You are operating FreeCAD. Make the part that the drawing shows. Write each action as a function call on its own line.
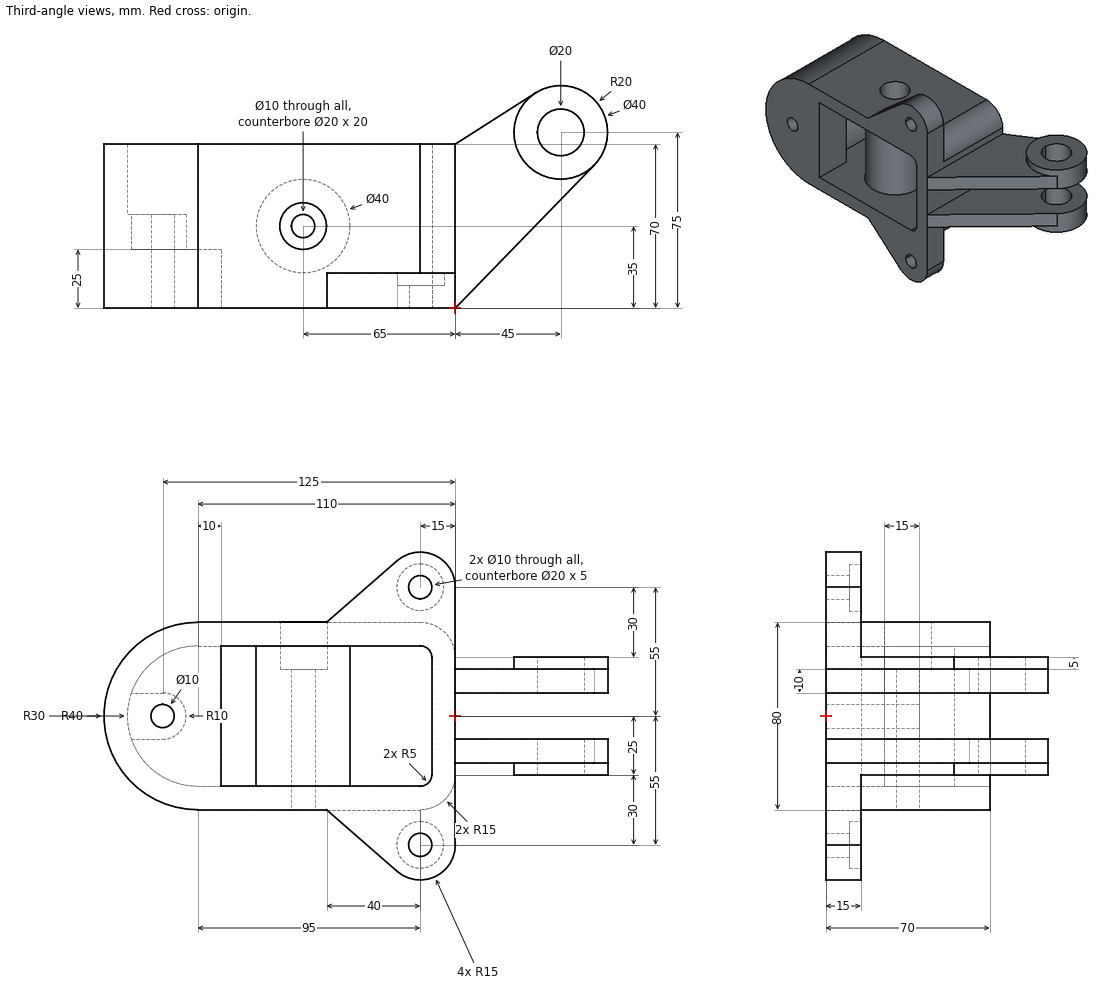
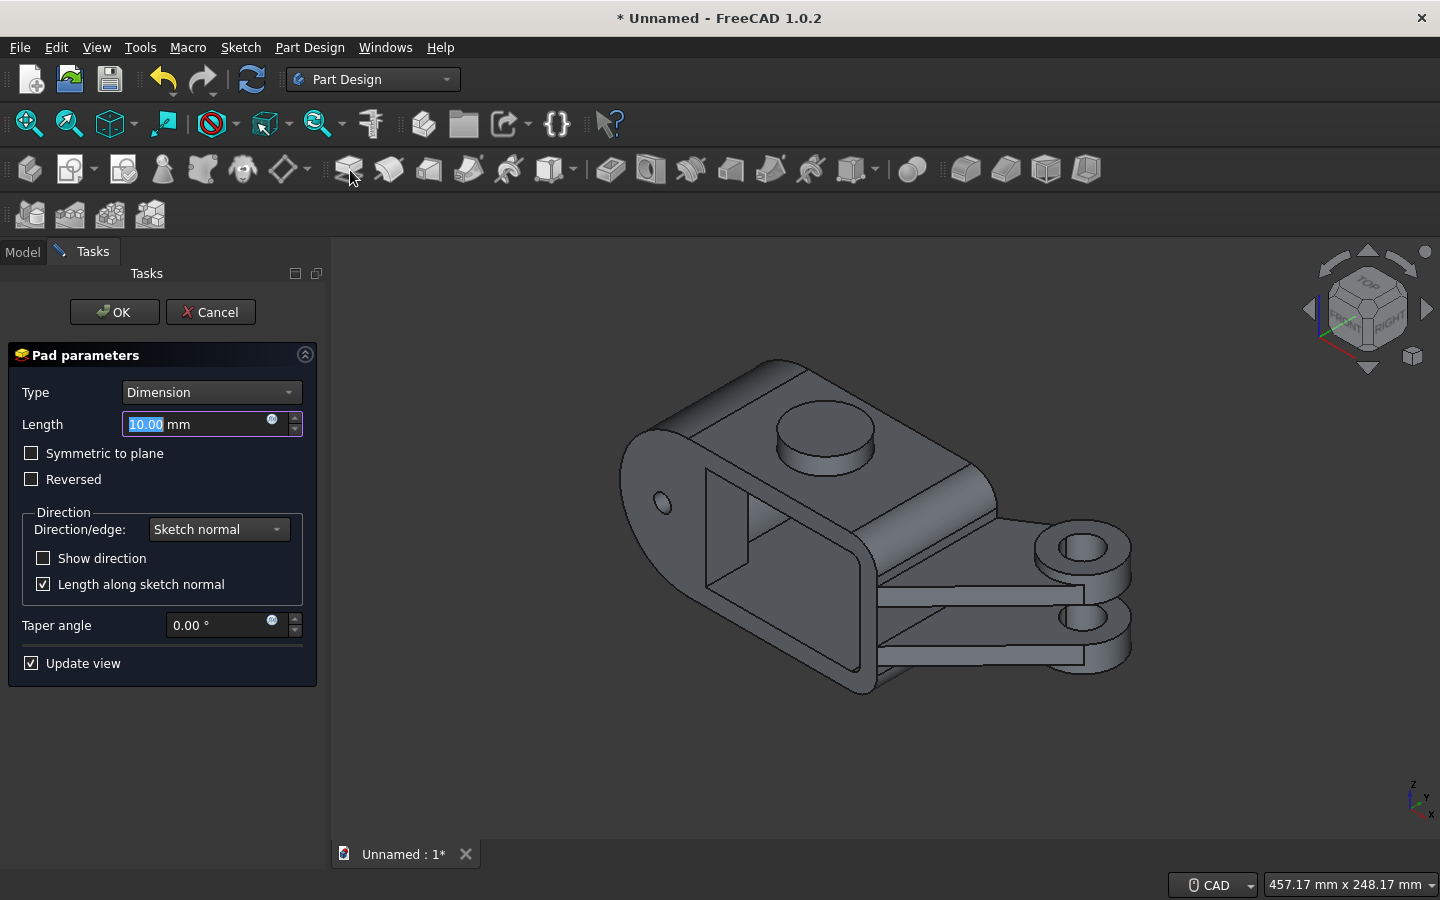
text(80)
key(Tab)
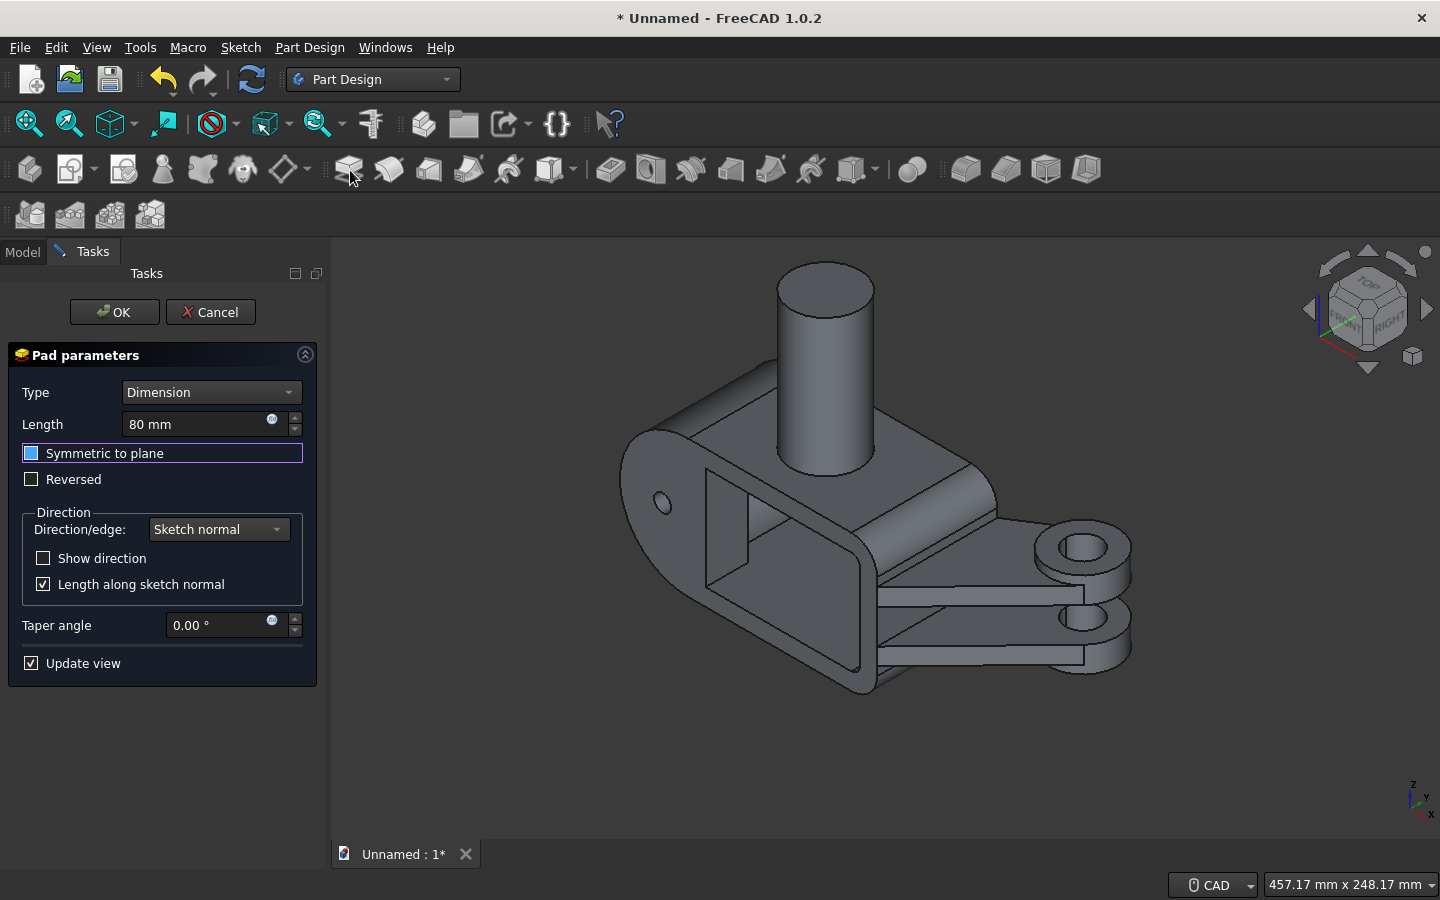
click(30, 479)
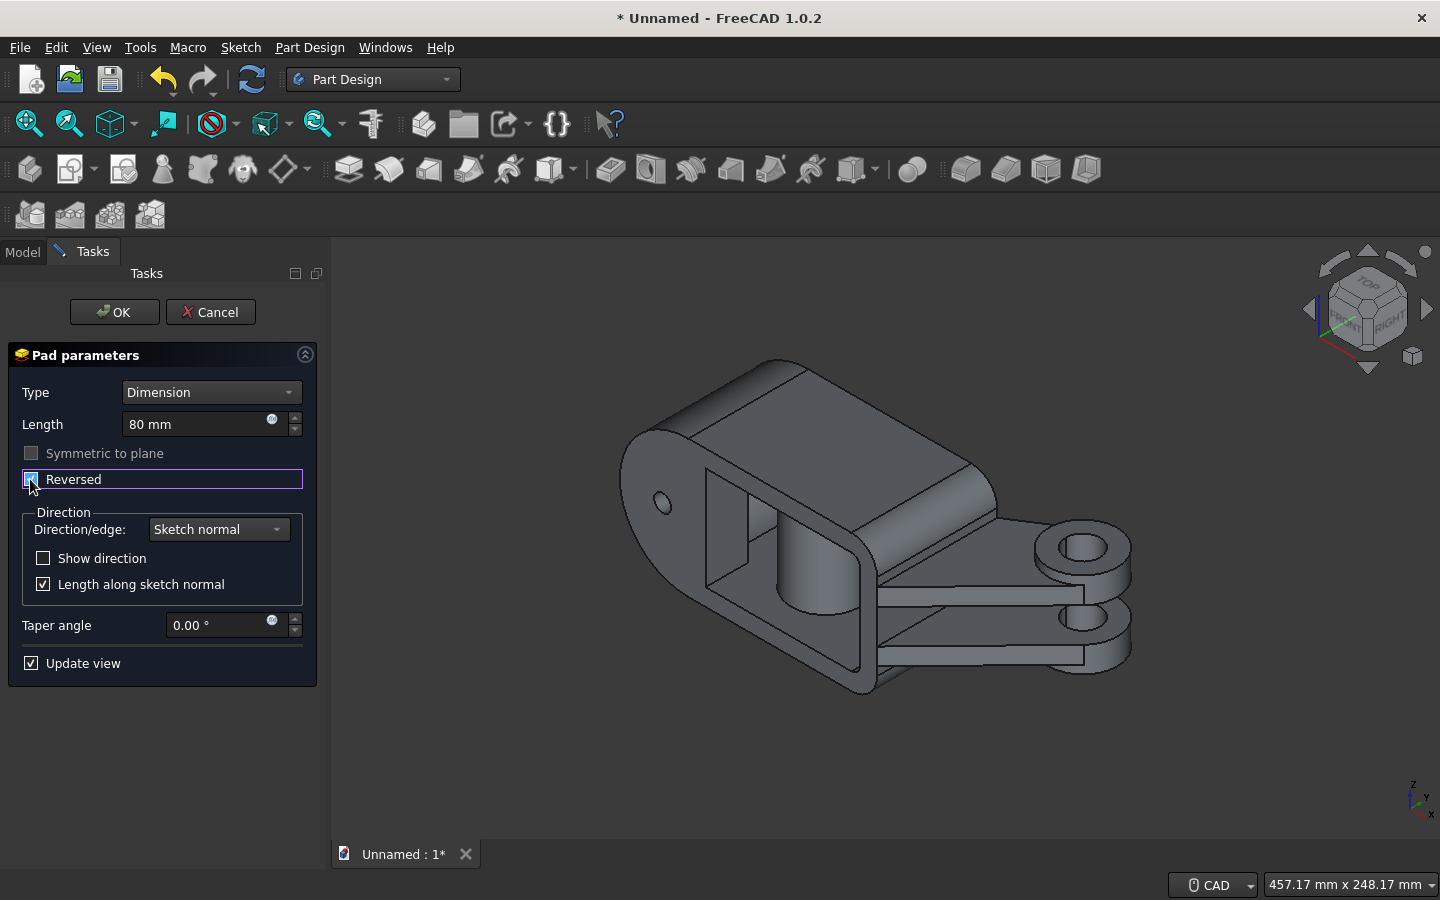
click(115, 312)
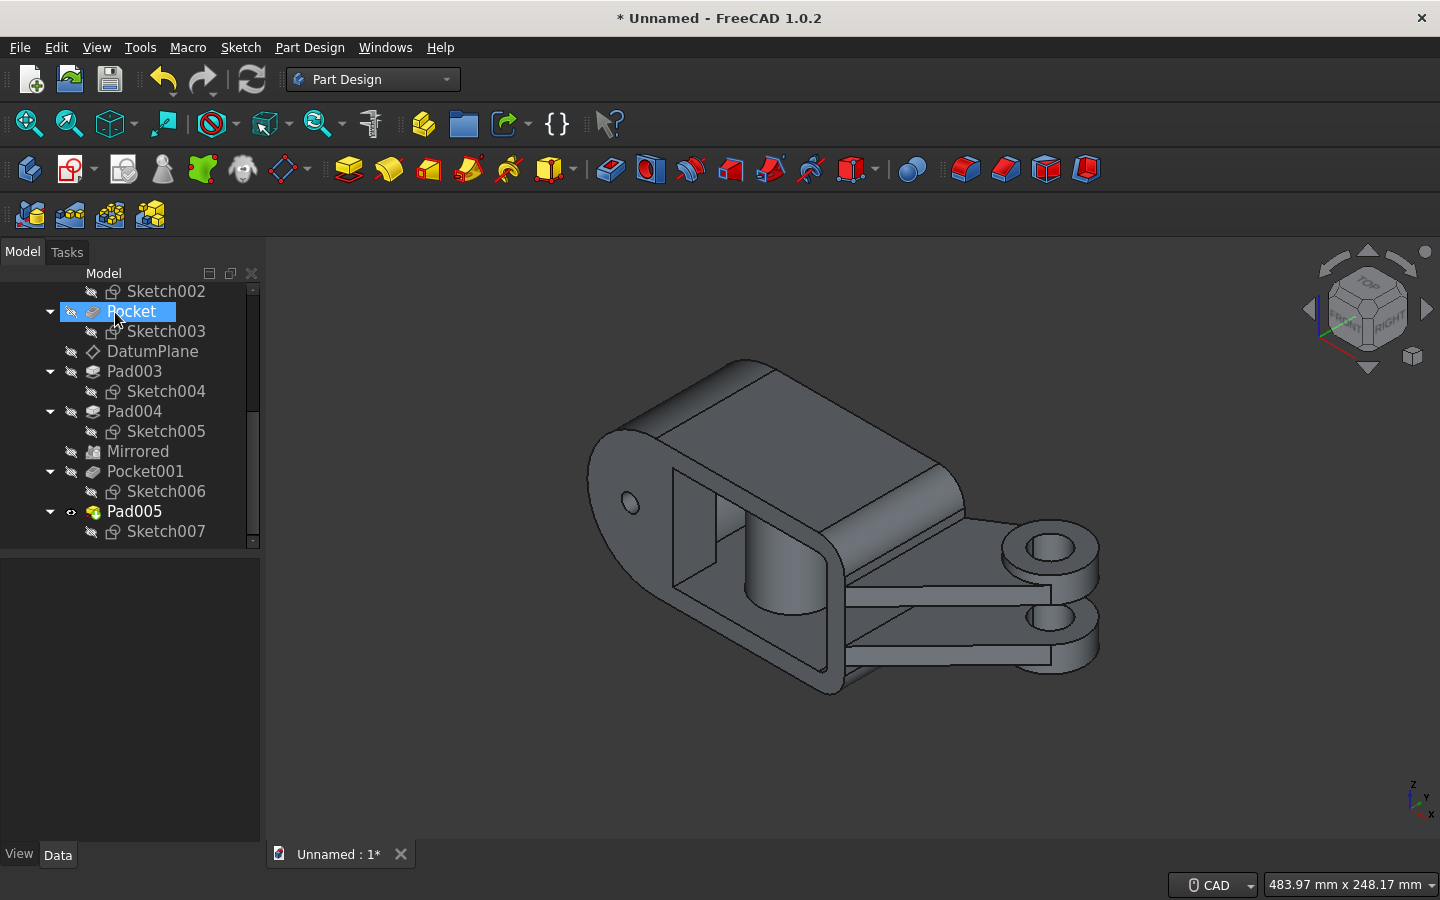
click(797, 450)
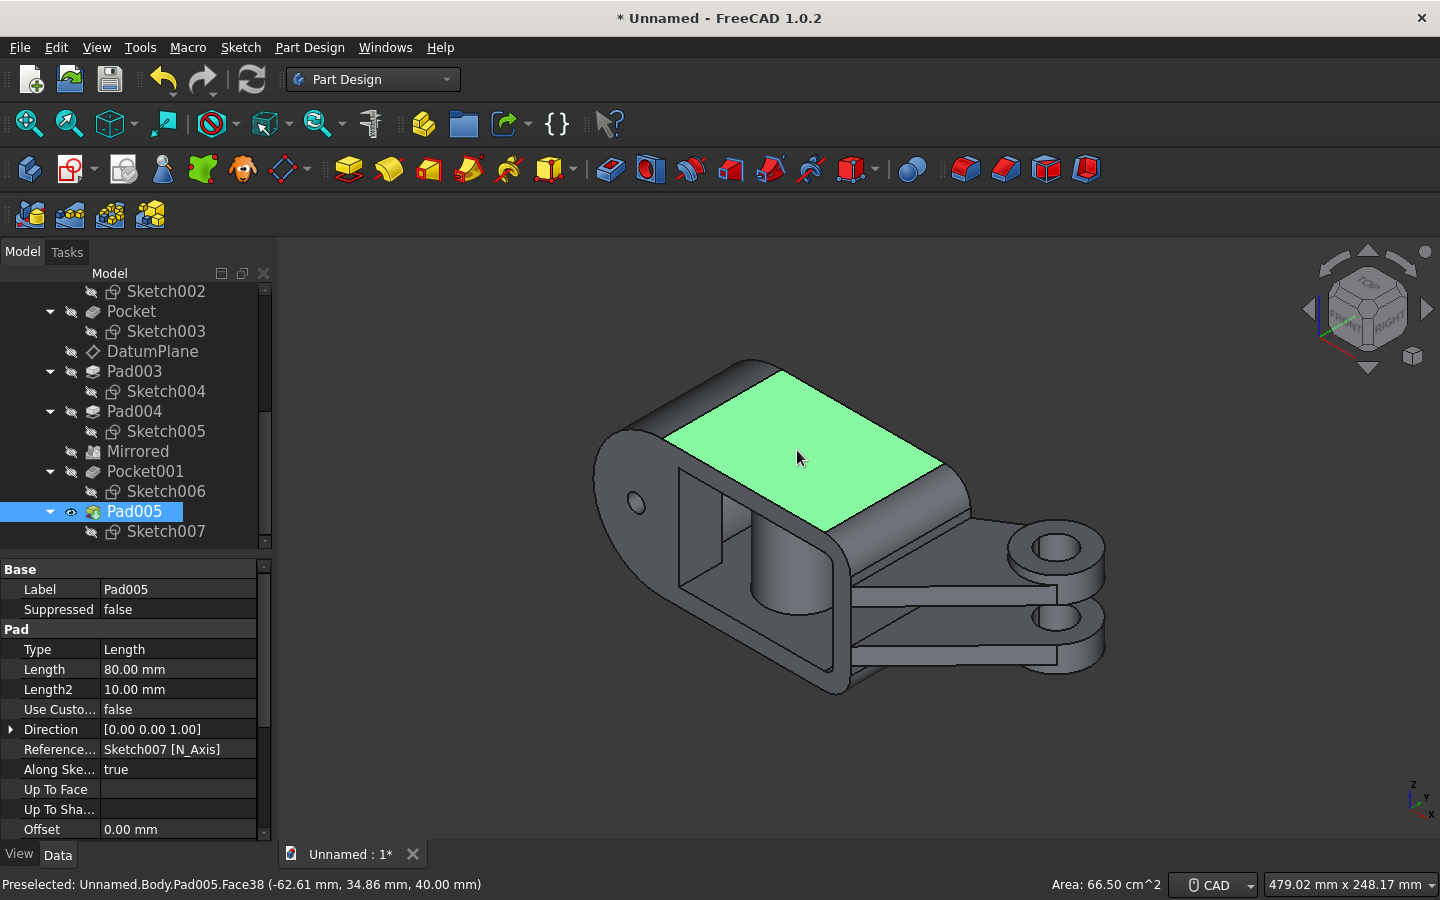
click(70, 170)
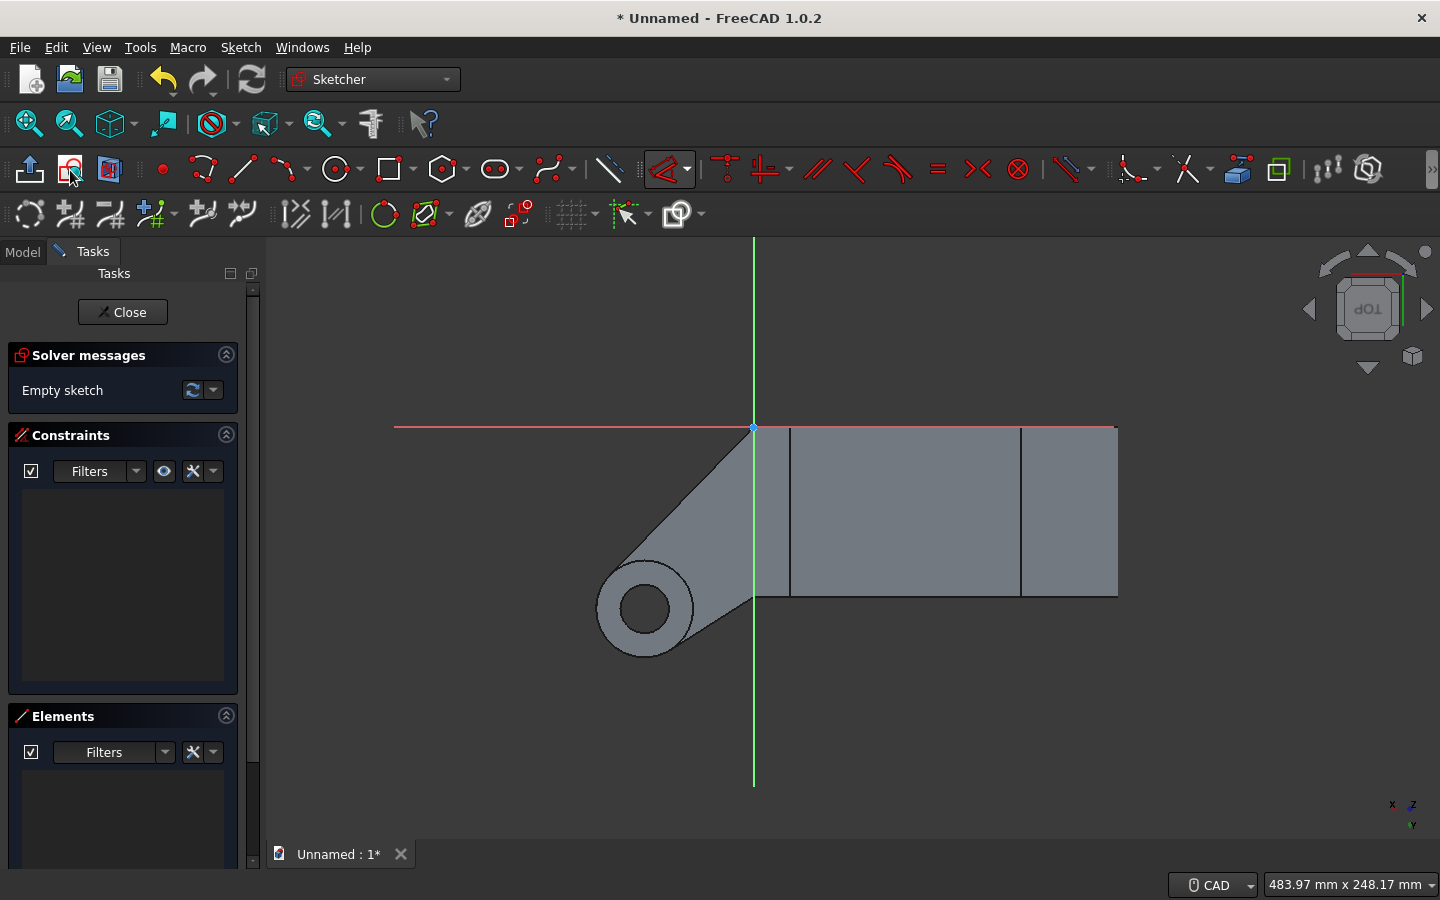
scroll(920, 510, up, 14)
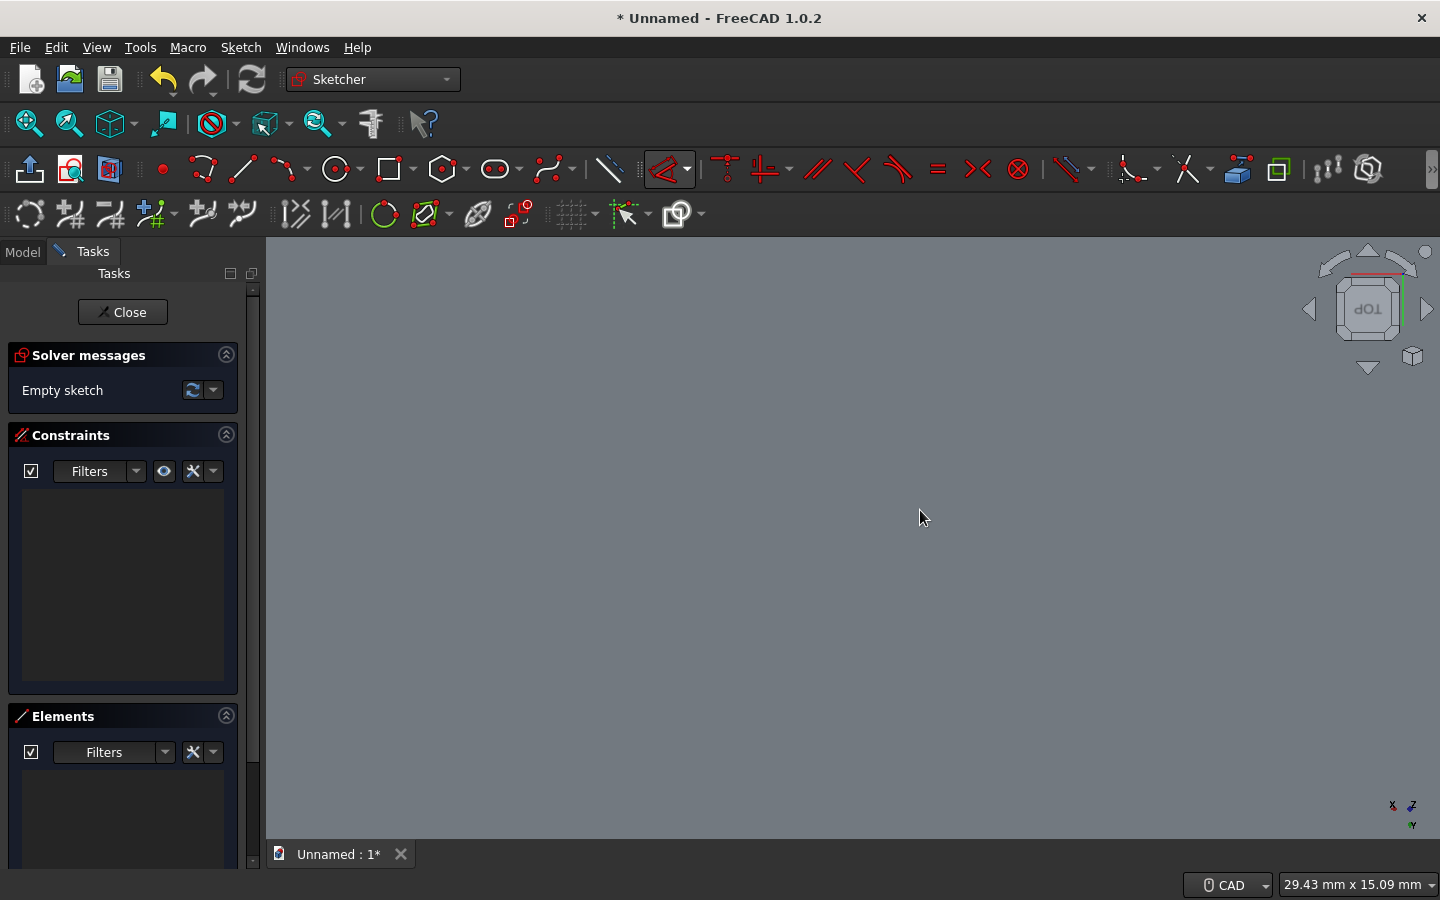
click(336, 170)